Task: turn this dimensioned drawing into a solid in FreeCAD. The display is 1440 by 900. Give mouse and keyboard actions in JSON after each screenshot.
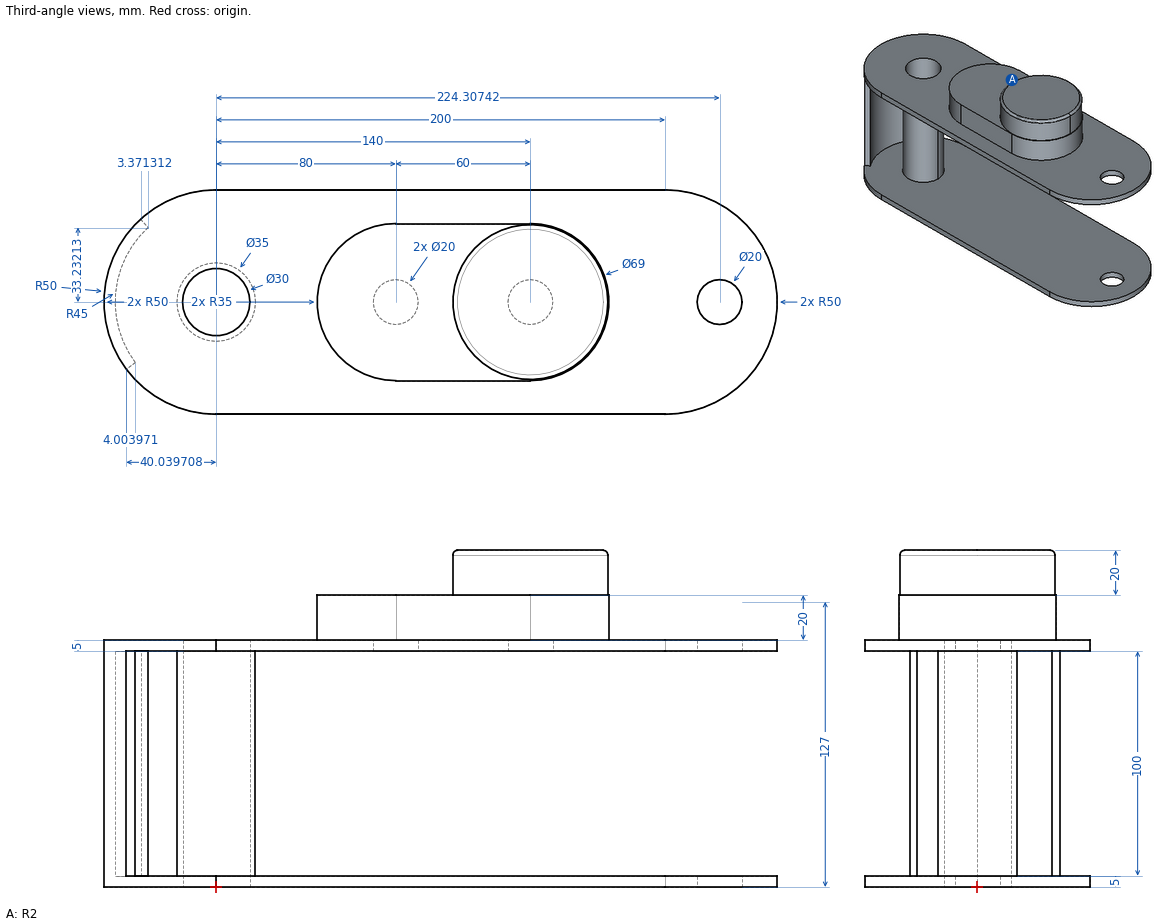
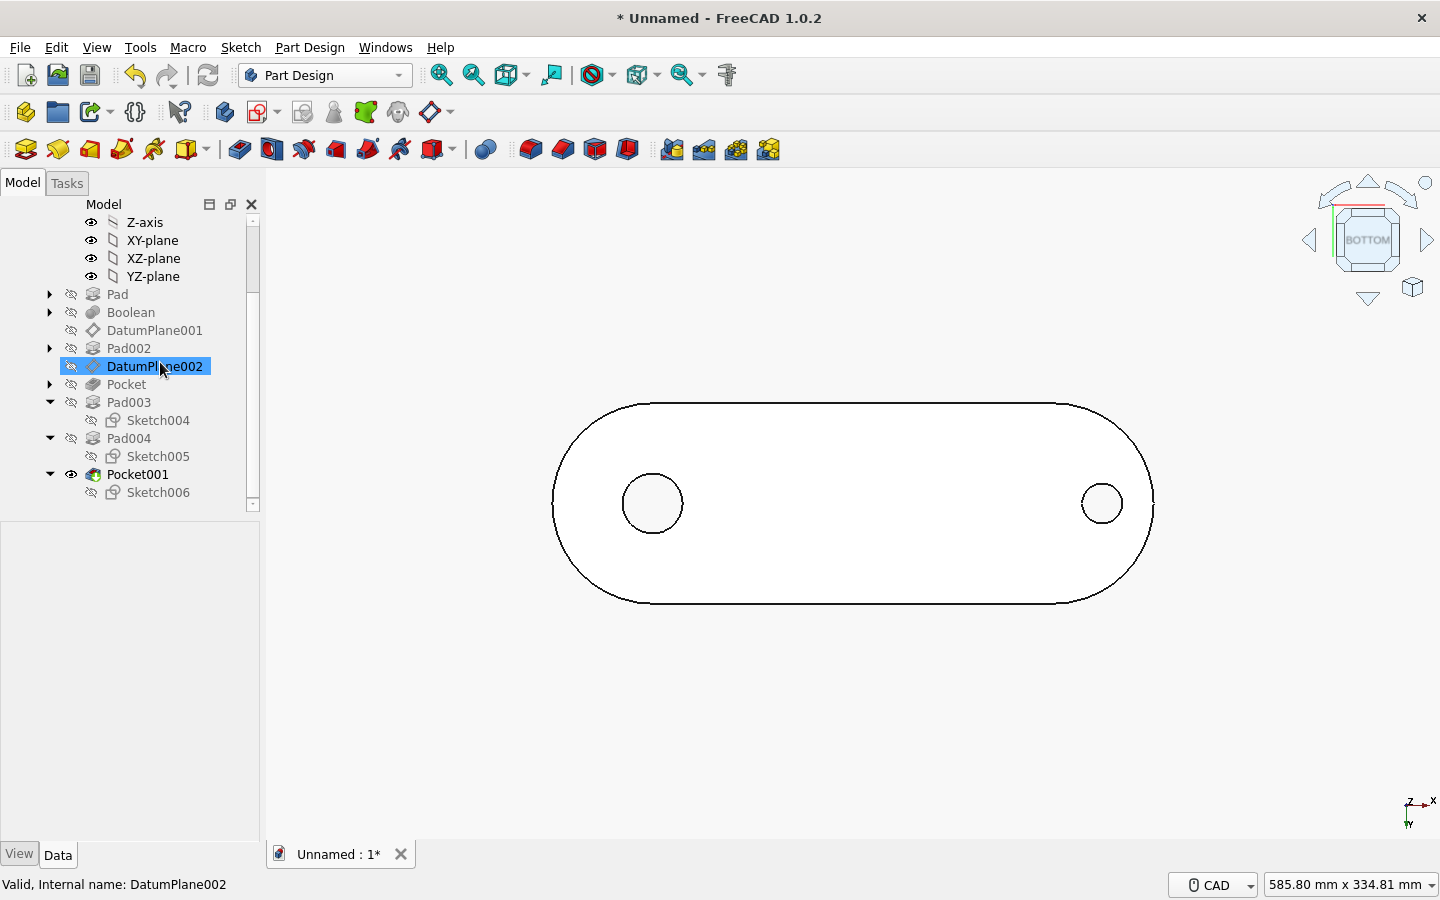
{"action": "scroll", "coordinate": [160, 362], "scroll_direction": "up", "scroll_amount": 15}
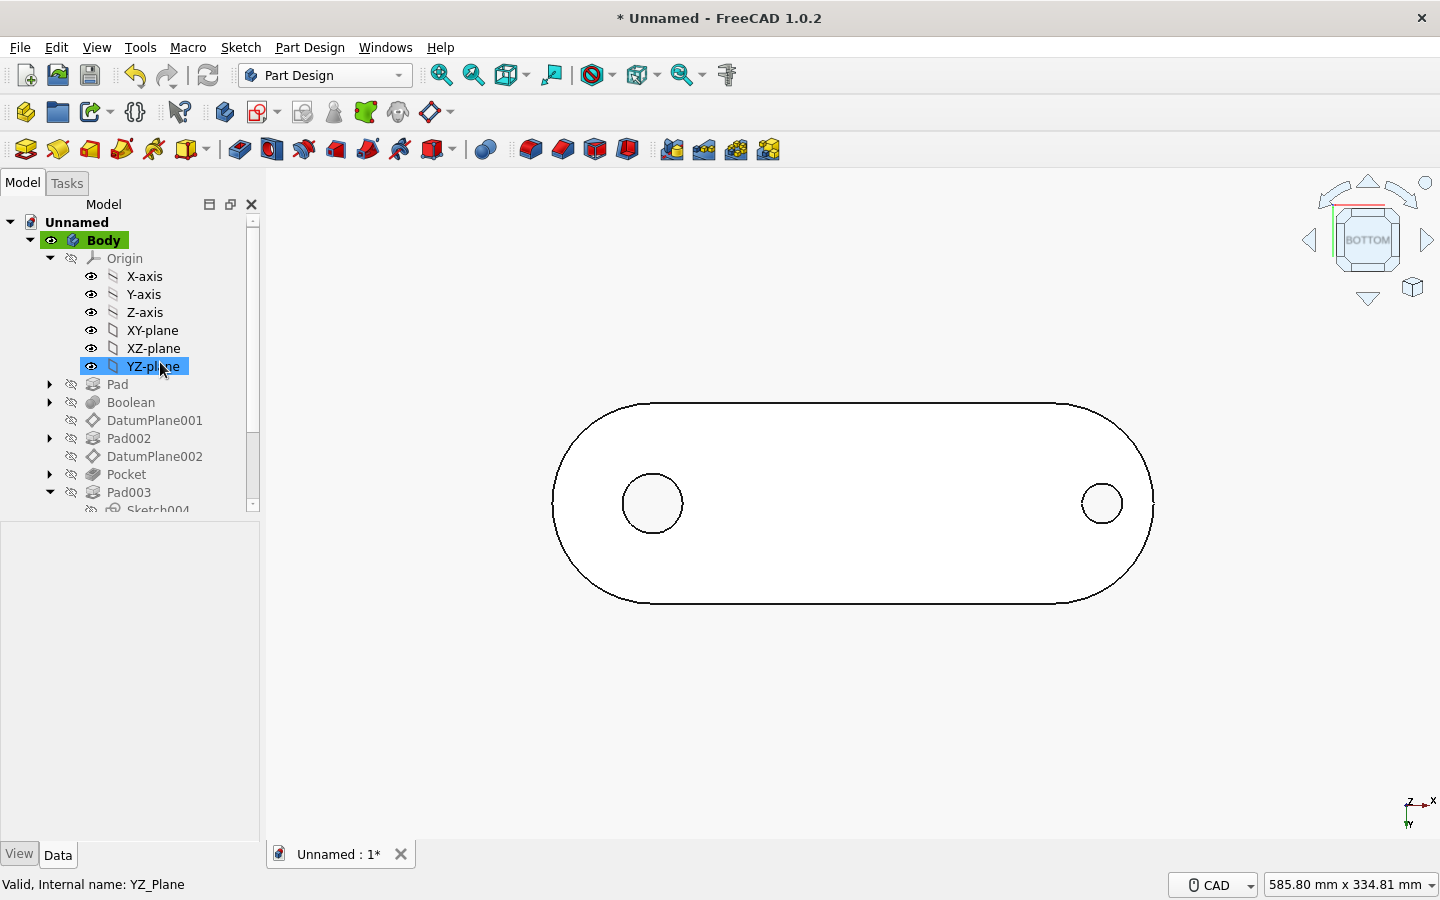
{"action": "left_click", "coordinate": [136, 330]}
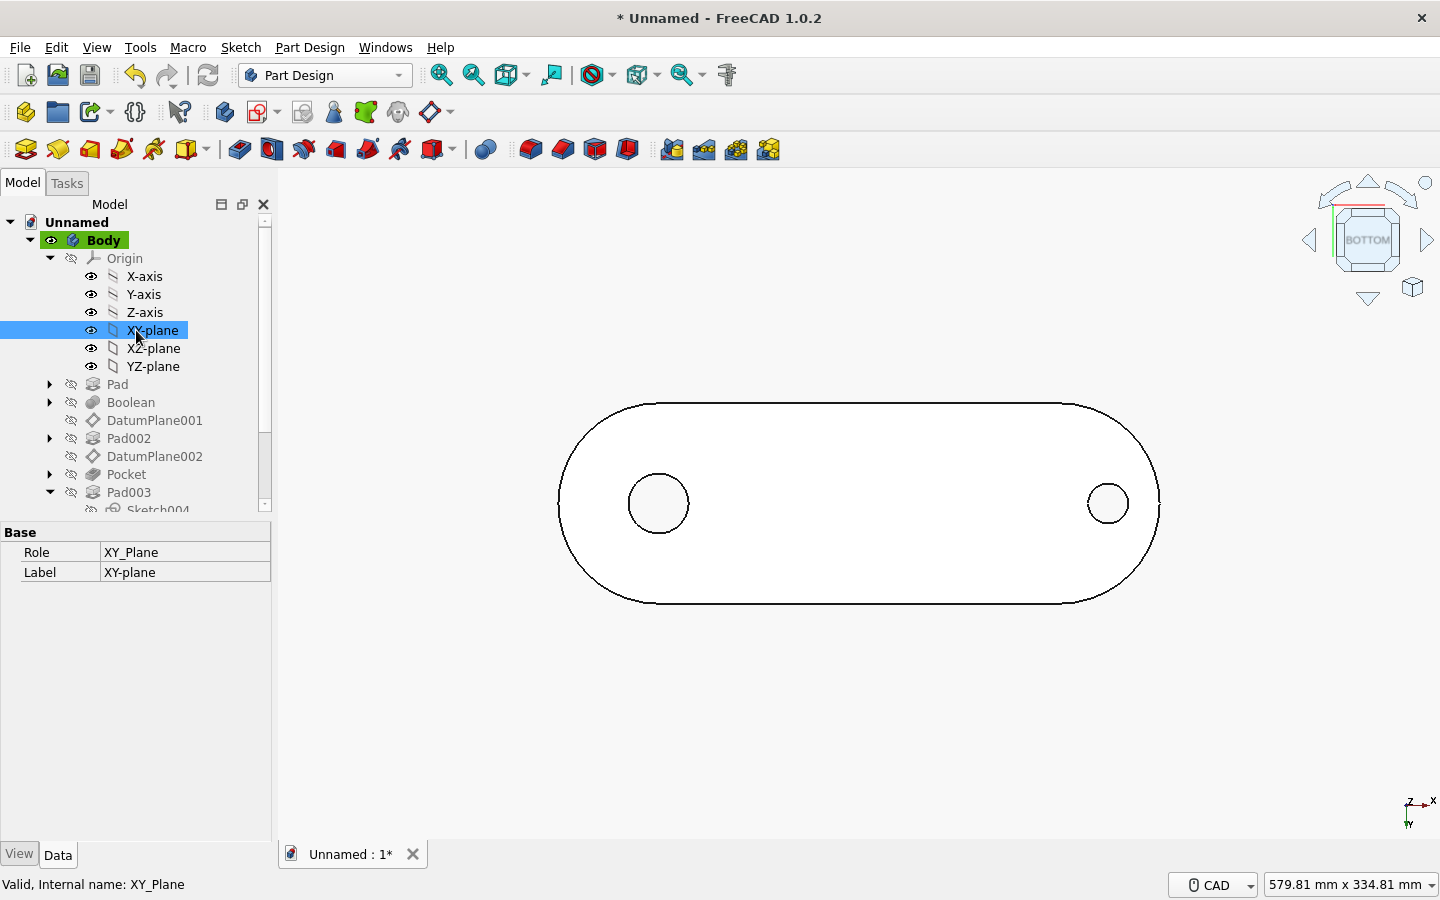
{"action": "left_click", "coordinate": [430, 112]}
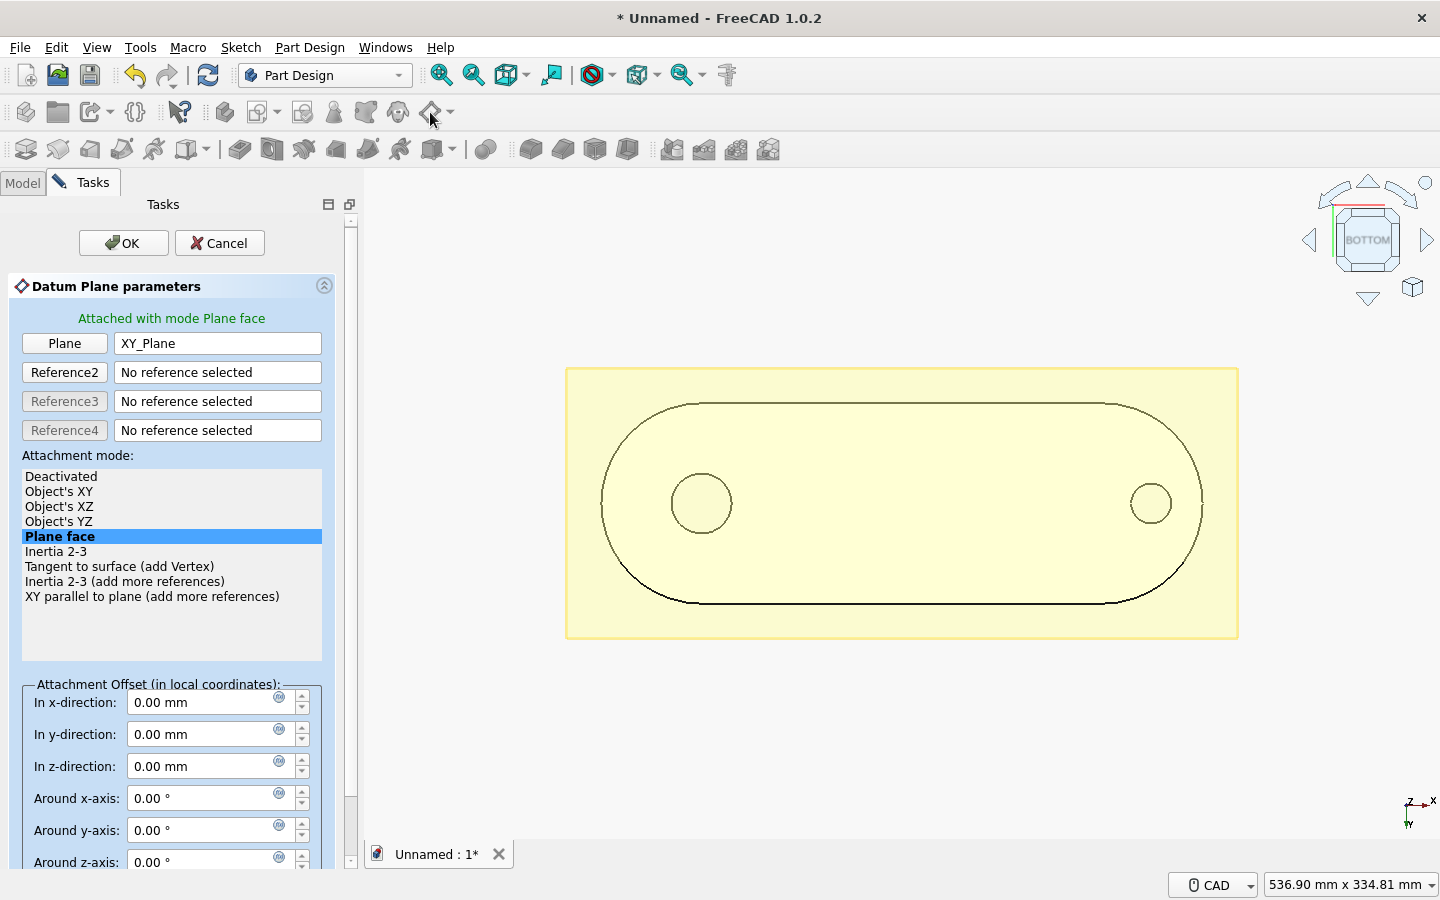
{"action": "triple_click", "coordinate": [210, 766]}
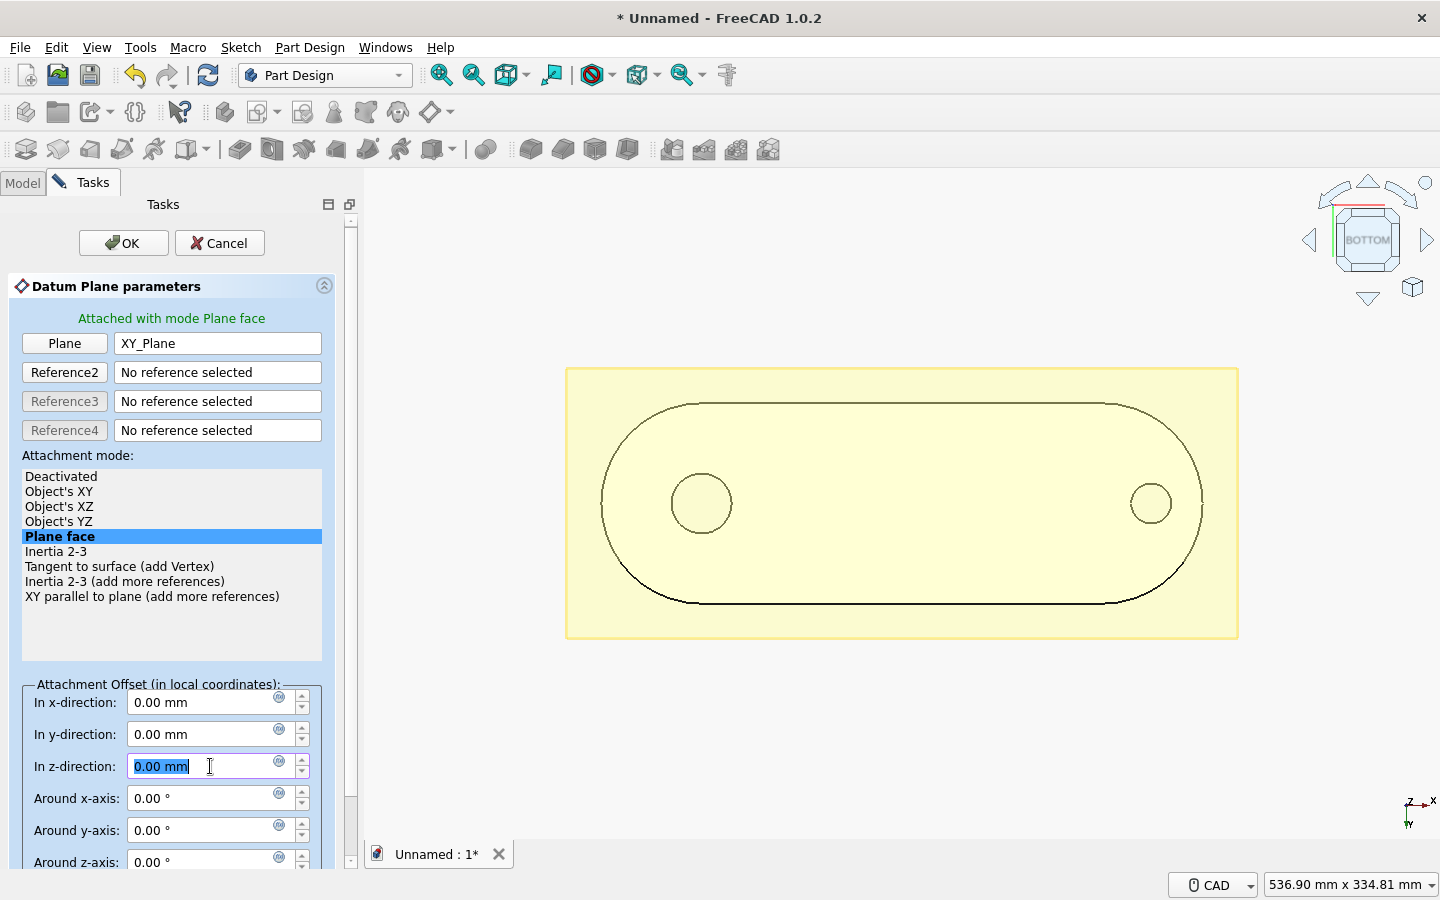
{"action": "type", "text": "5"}
{"action": "key", "text": "Tab"}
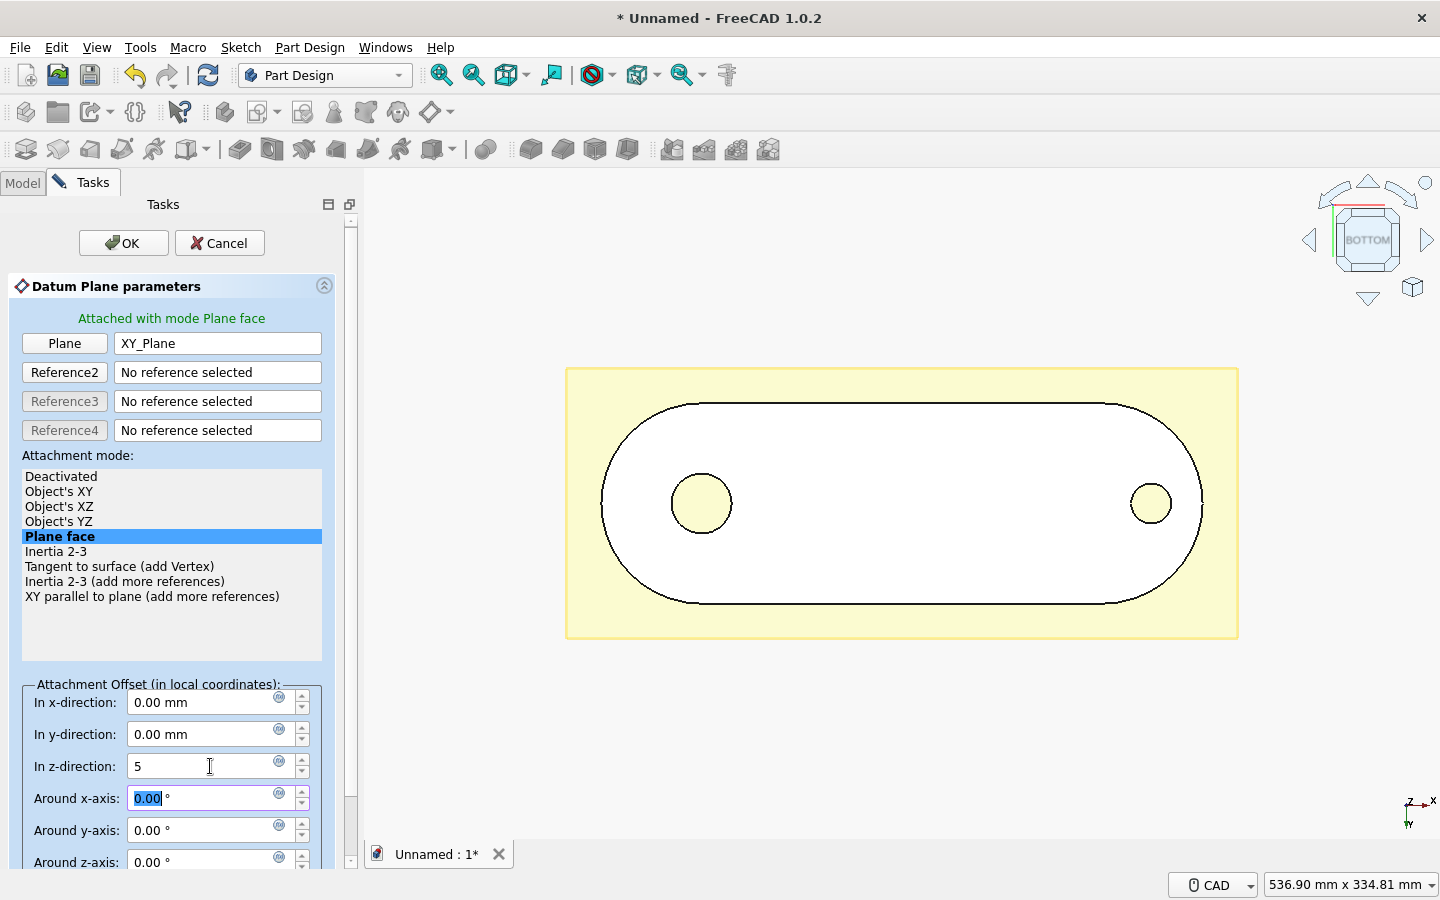
{"action": "left_click", "coordinate": [124, 243]}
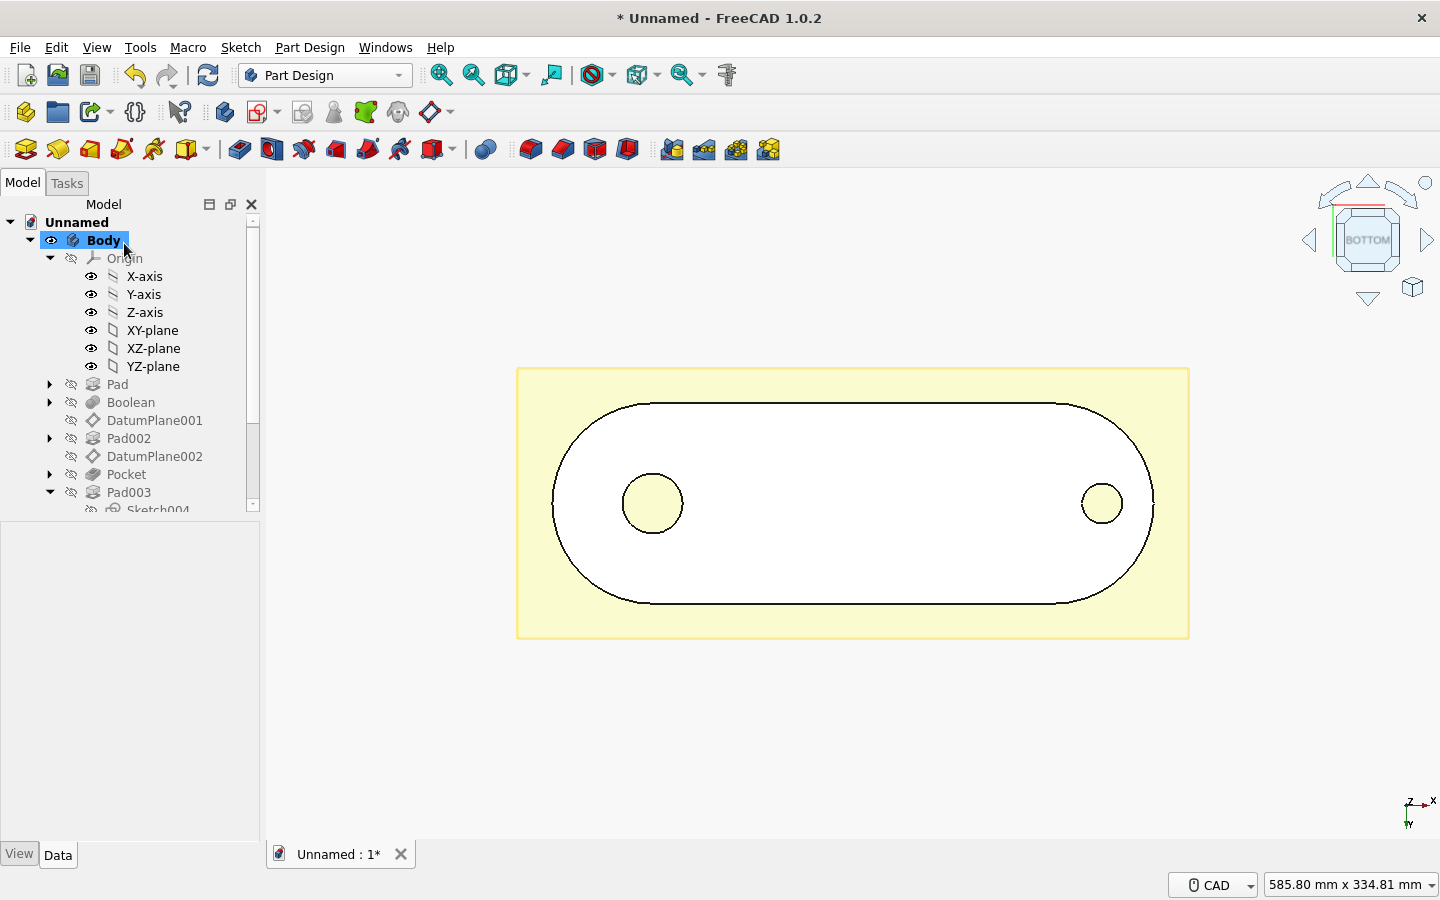
{"action": "scroll", "coordinate": [100, 362], "scroll_direction": "down", "scroll_amount": 3}